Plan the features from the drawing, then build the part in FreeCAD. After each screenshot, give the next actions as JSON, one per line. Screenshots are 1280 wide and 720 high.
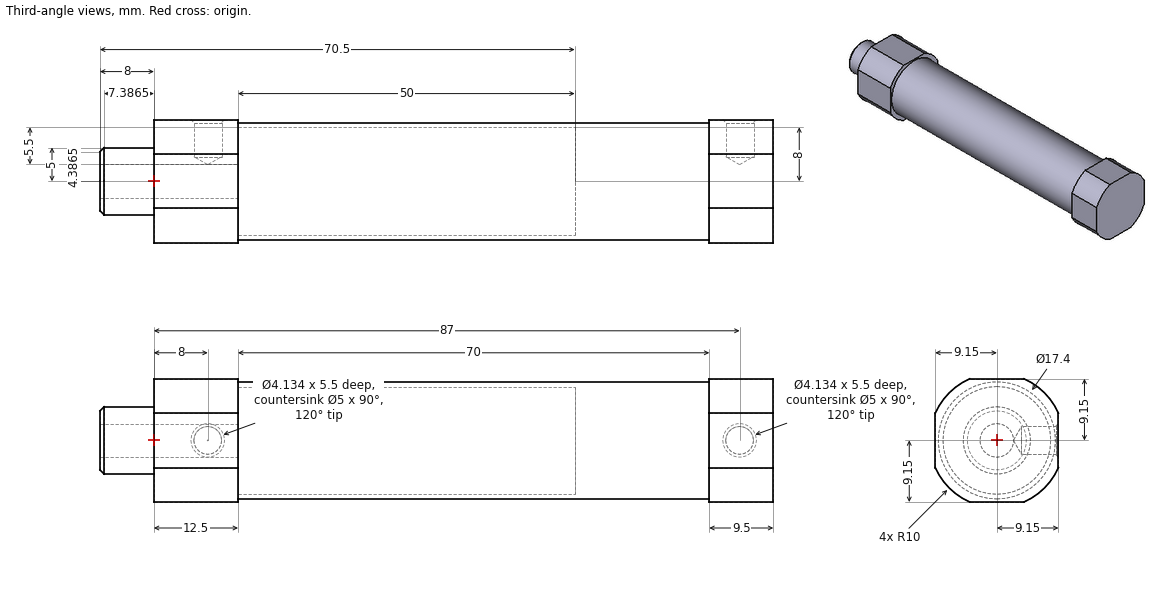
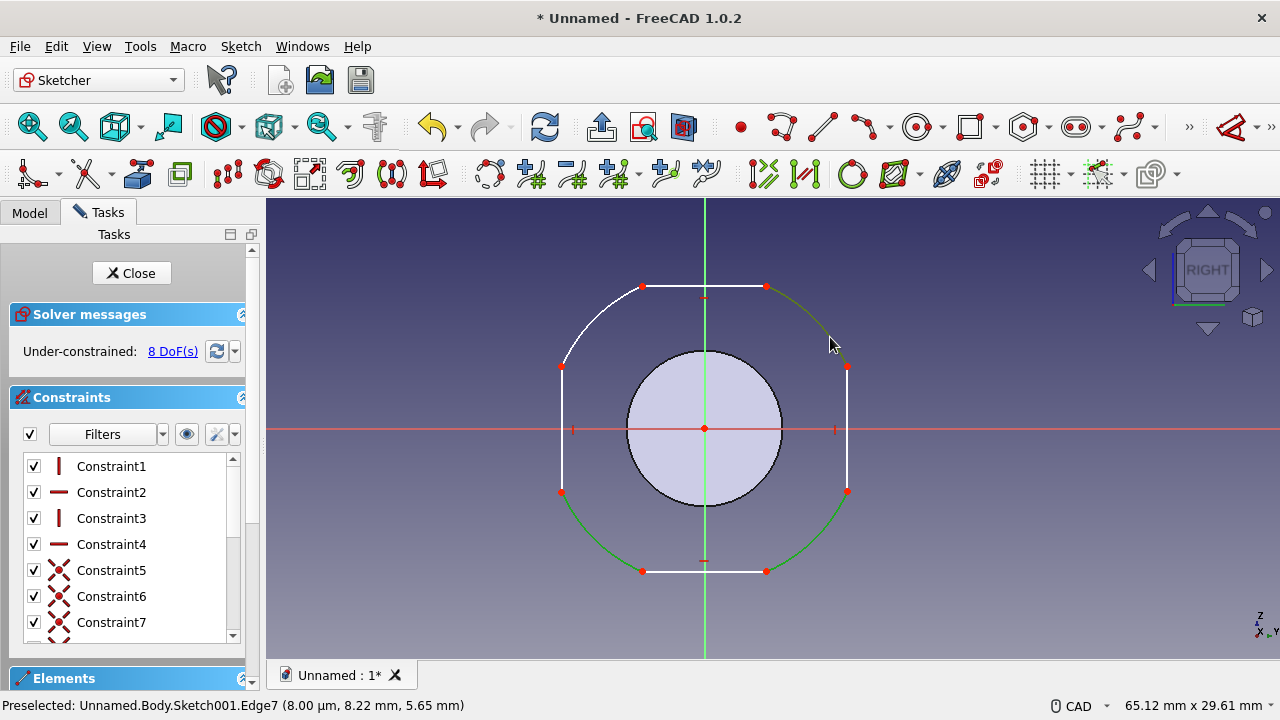
{"action": "left_click", "coordinate": [612, 304]}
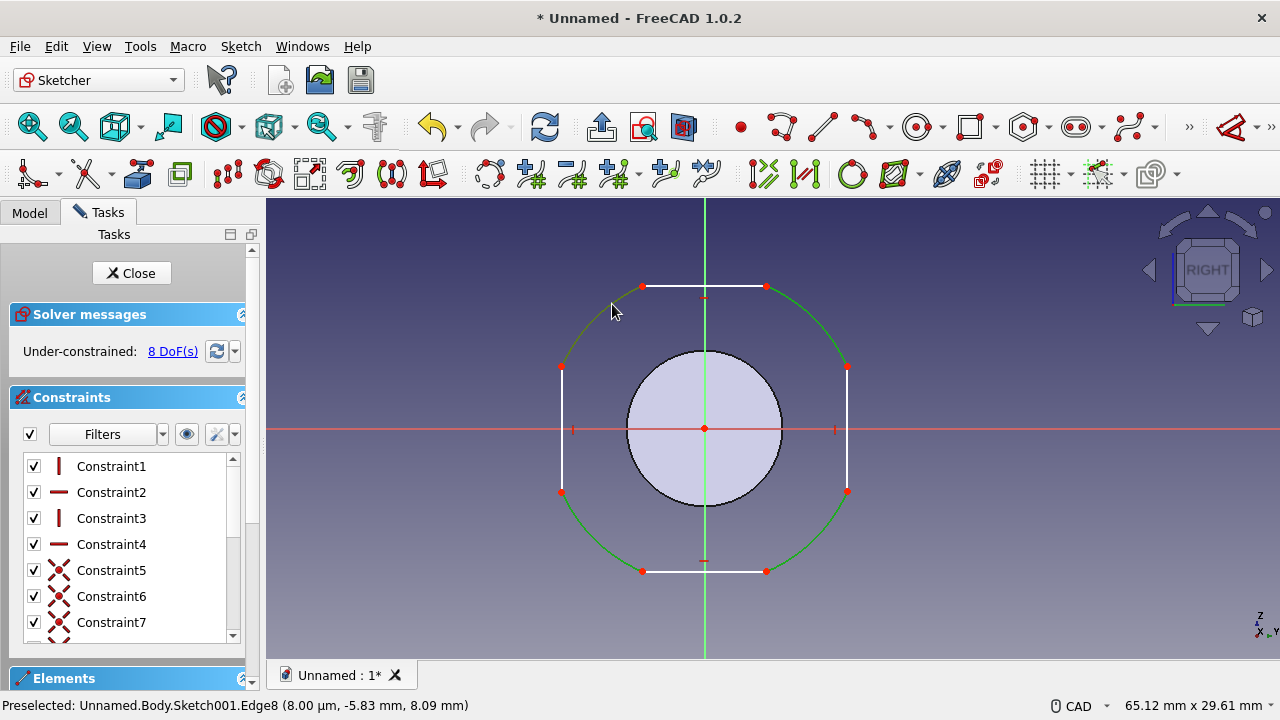
{"action": "key", "text": "e"}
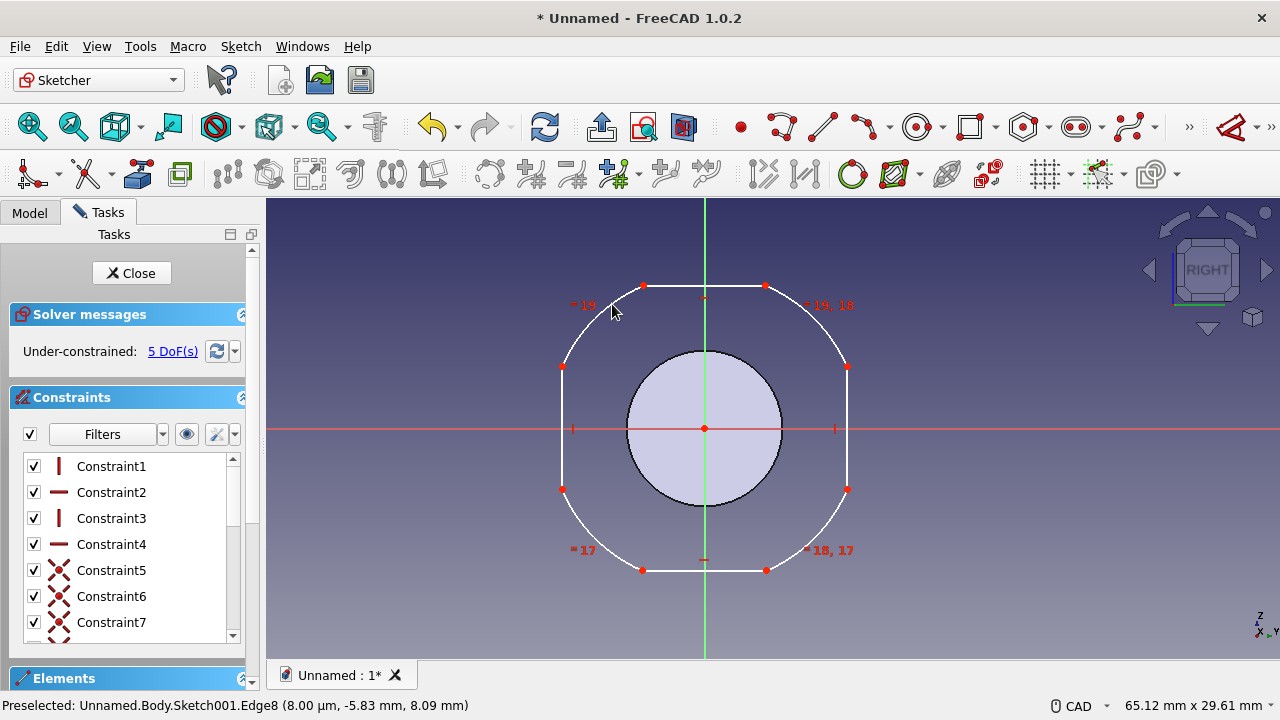
{"action": "left_click", "coordinate": [1230, 128]}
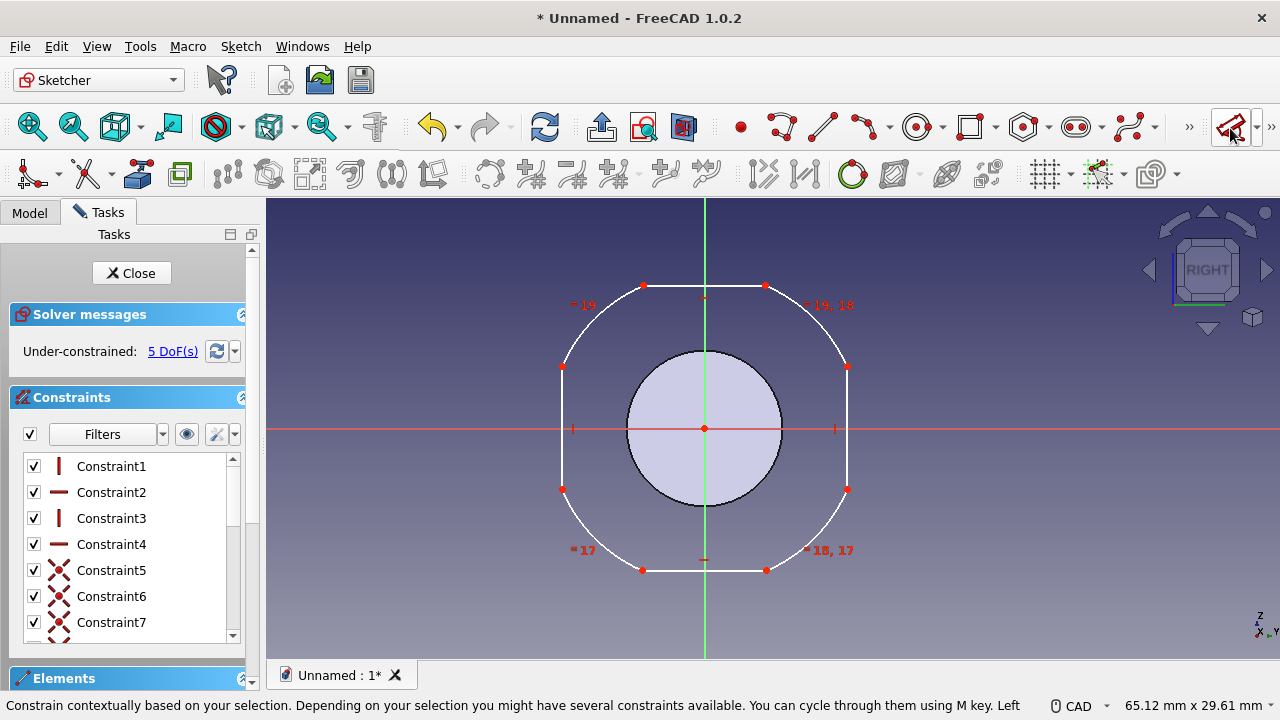
{"action": "left_click", "coordinate": [579, 520]}
{"action": "left_click", "coordinate": [553, 539]}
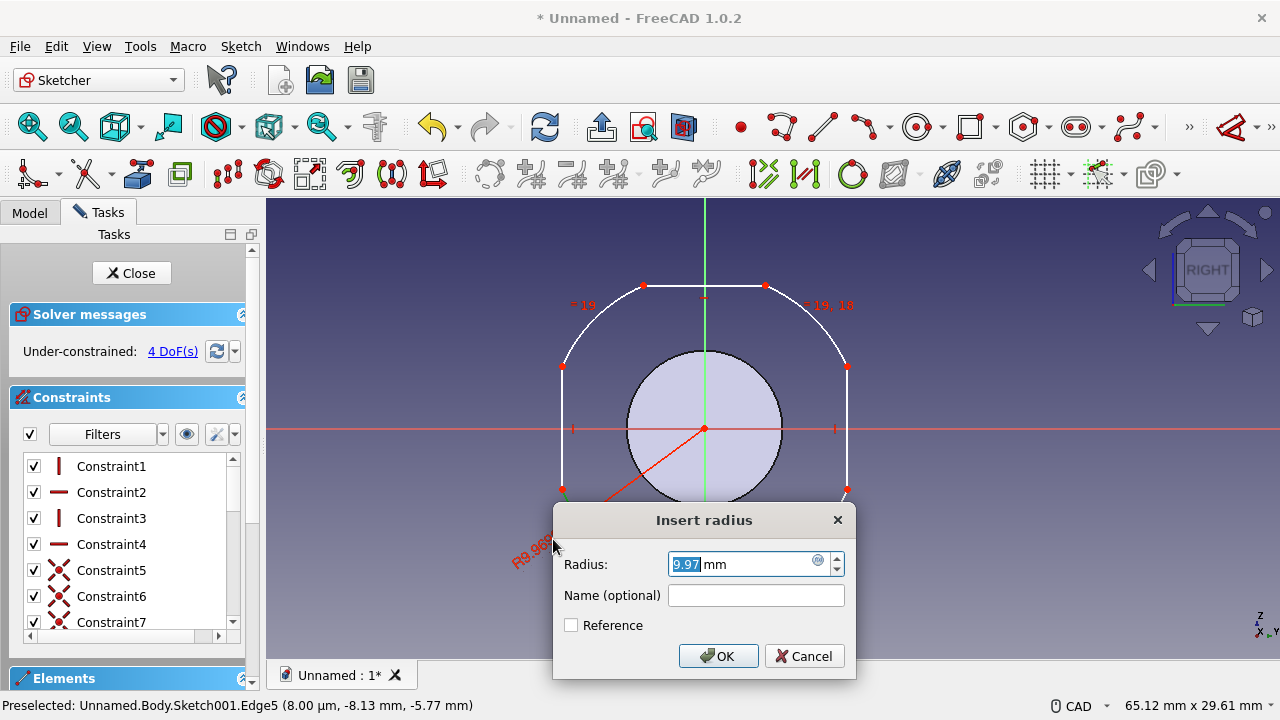
{"action": "type", "text": "10"}
{"action": "key", "text": "Return"}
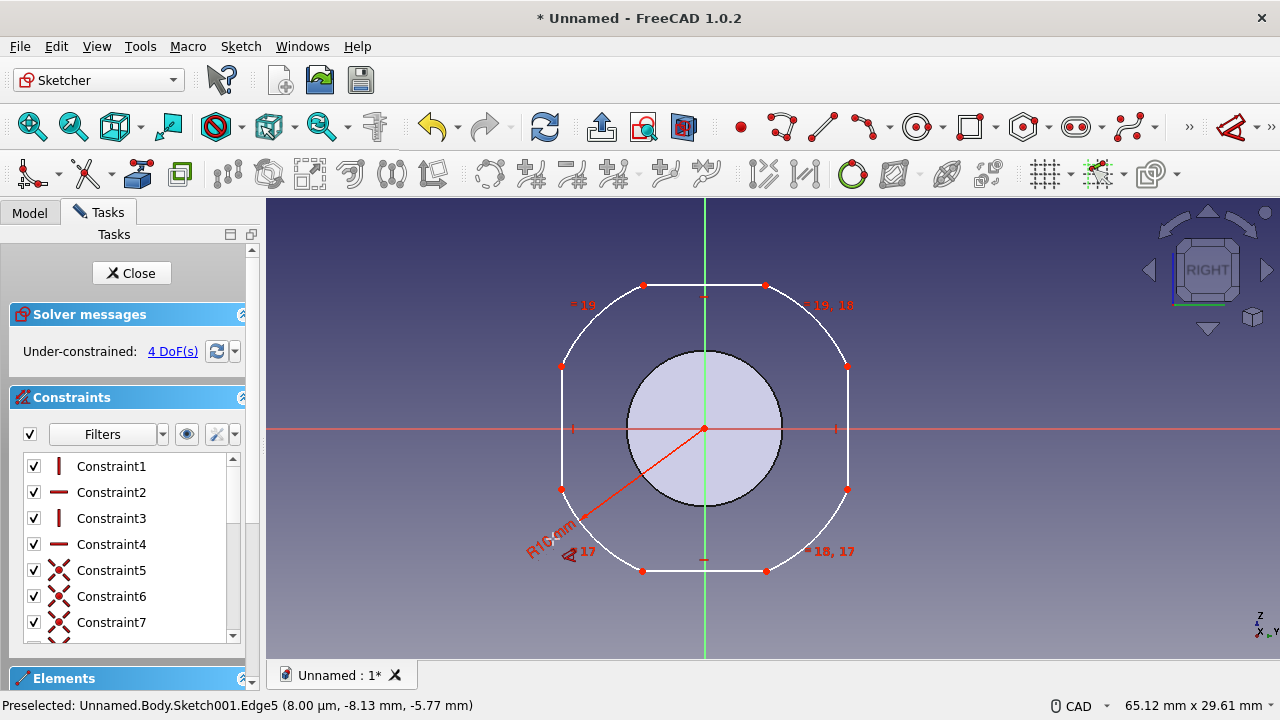
{"action": "left_click", "coordinate": [562, 367]}
{"action": "left_click", "coordinate": [633, 333]}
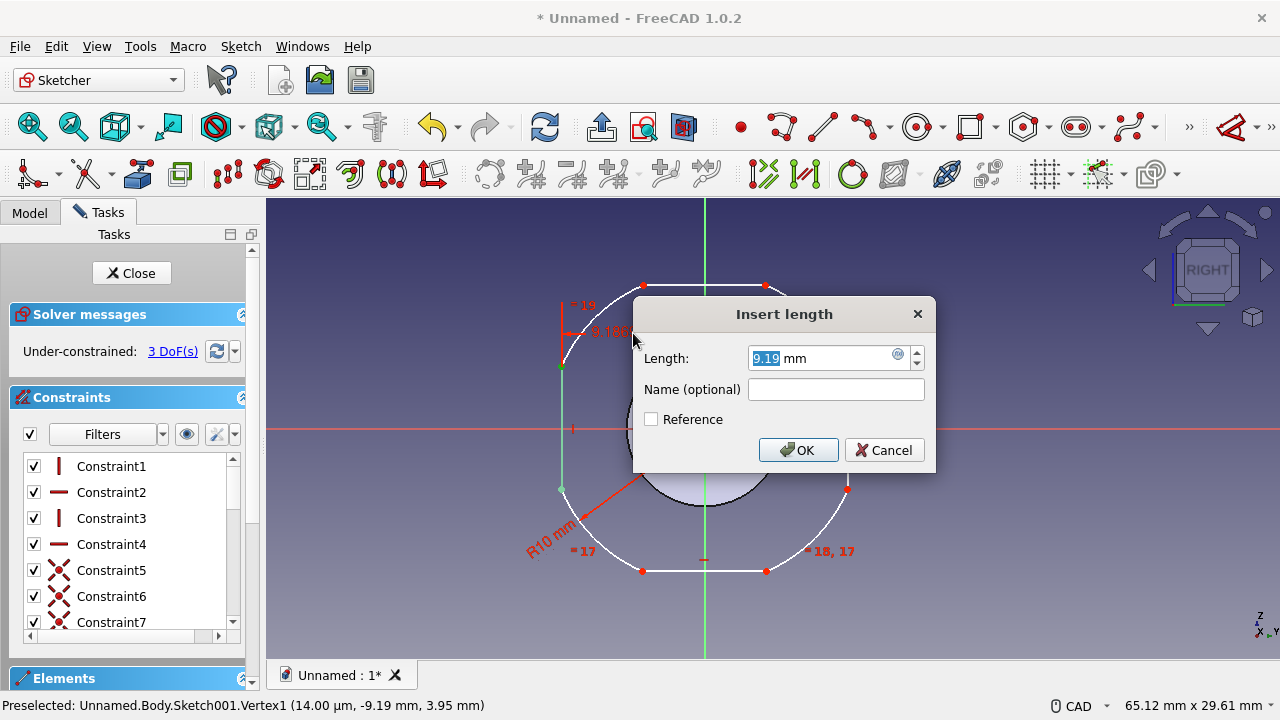
{"action": "type", "text": "9.15"}
{"action": "key", "text": "Return"}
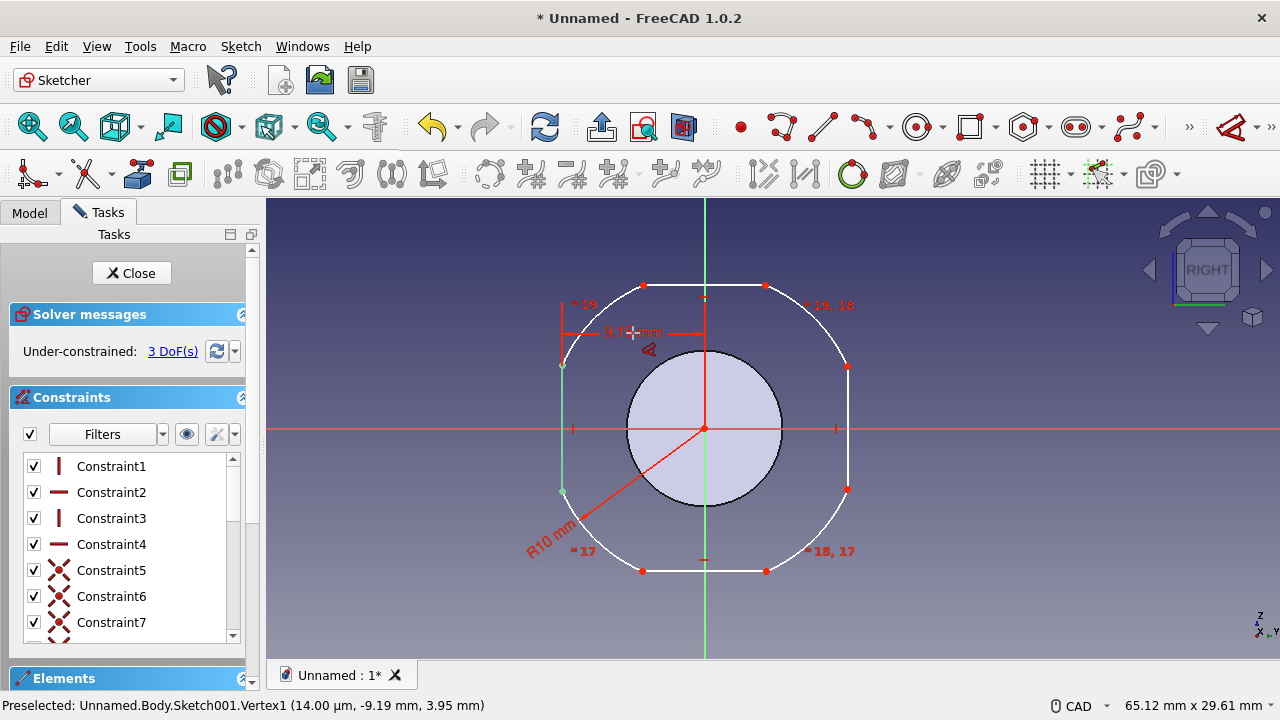
{"action": "left_click", "coordinate": [642, 571]}
{"action": "left_click", "coordinate": [608, 500]}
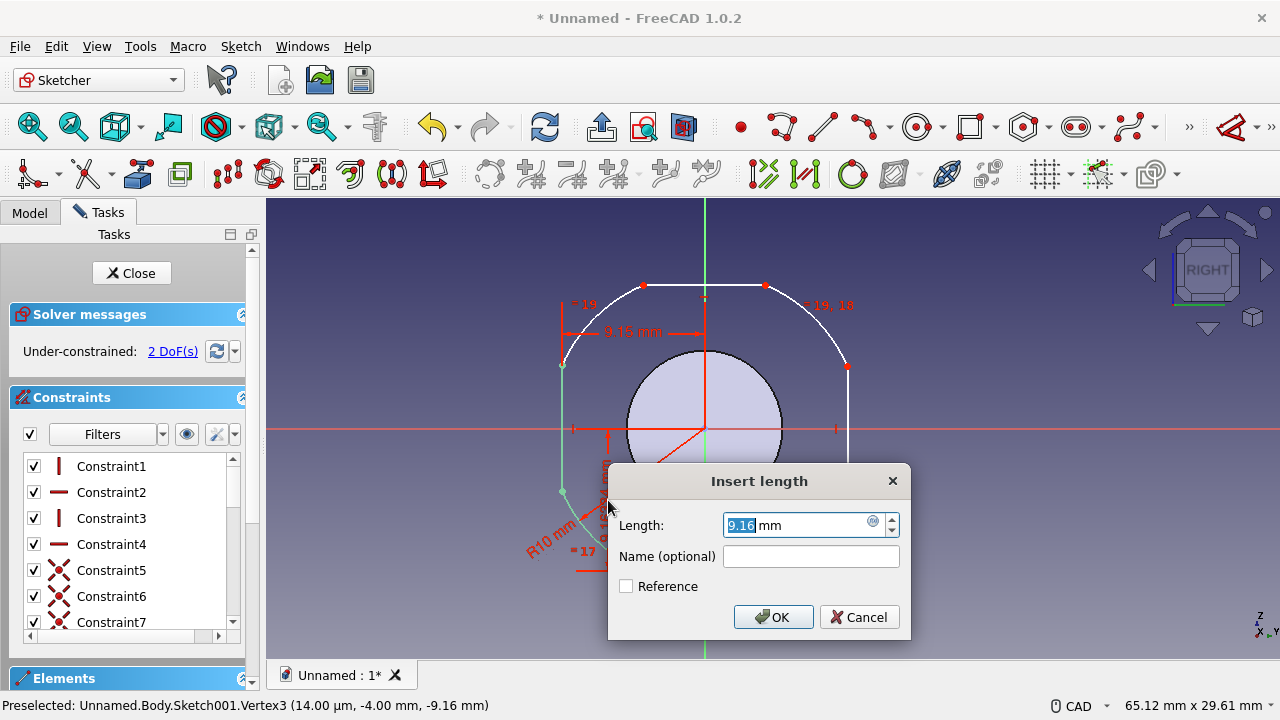
{"action": "type", "text": "9.15"}
{"action": "key", "text": "Return"}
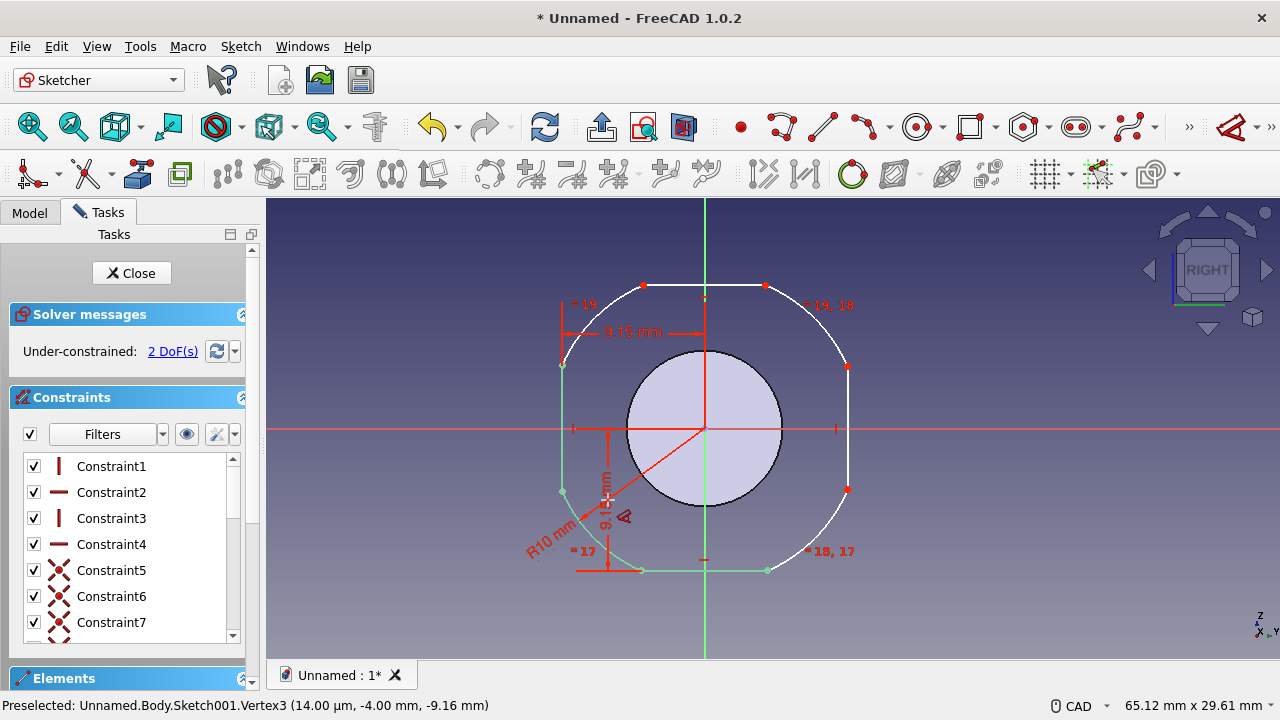
{"action": "left_click", "coordinate": [848, 490]}
{"action": "left_click", "coordinate": [776, 524]}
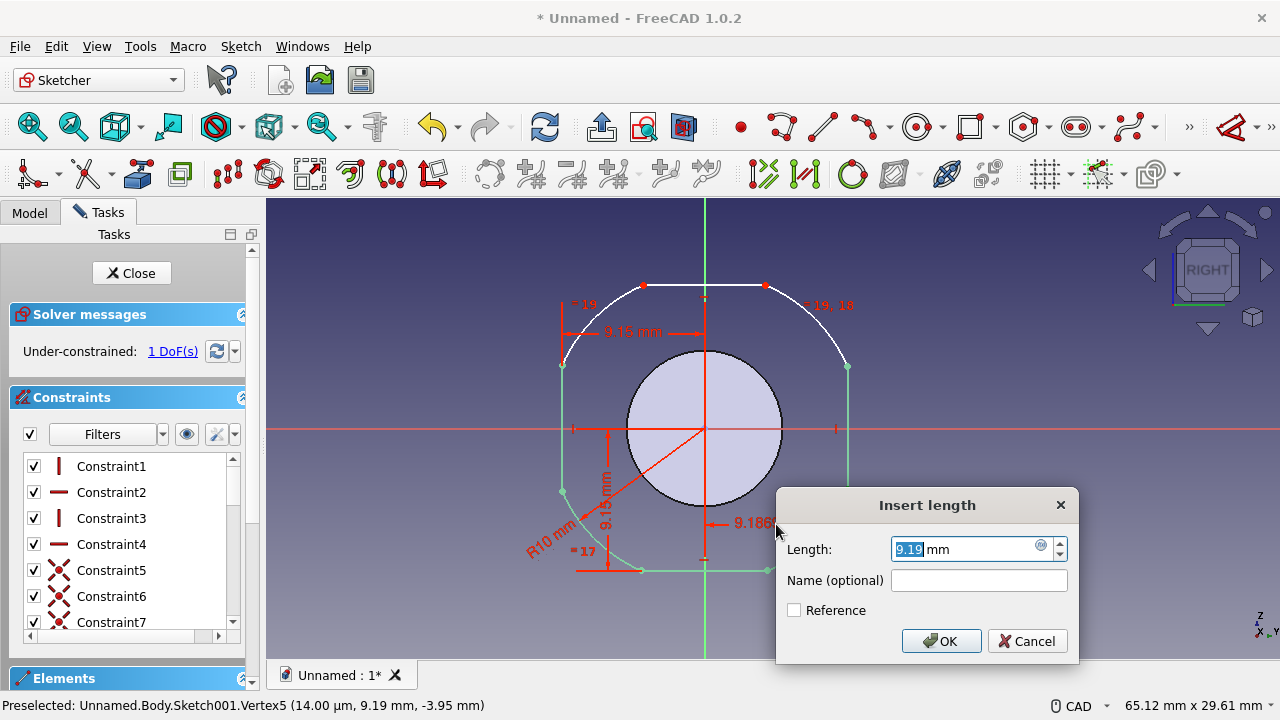
{"action": "type", "text": "9.15"}
{"action": "key", "text": "Return"}